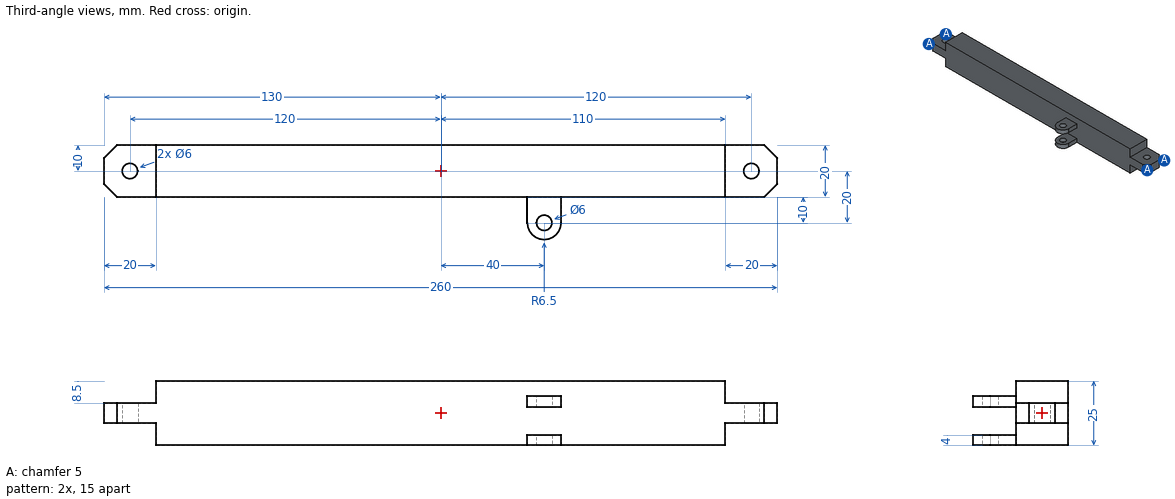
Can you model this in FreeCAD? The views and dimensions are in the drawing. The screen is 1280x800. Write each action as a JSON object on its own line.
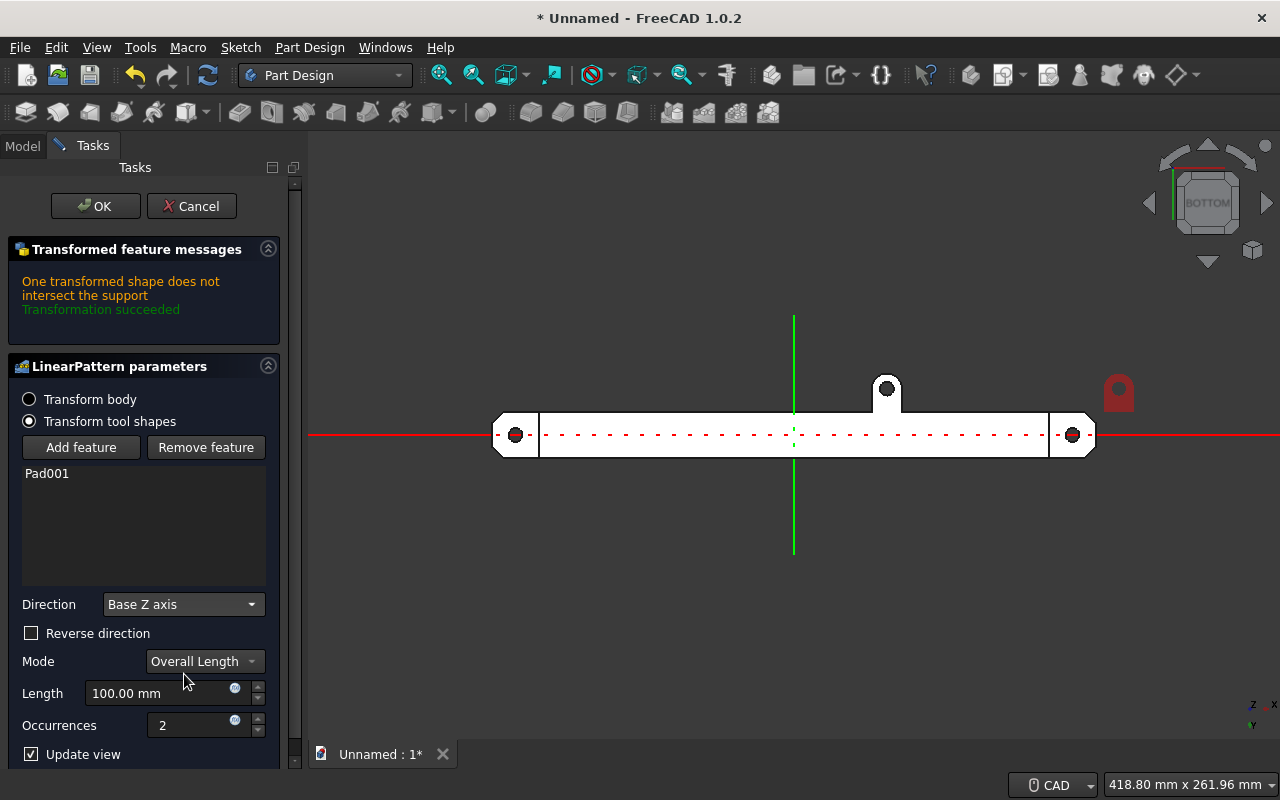
{"action": "left_click", "coordinate": [206, 662]}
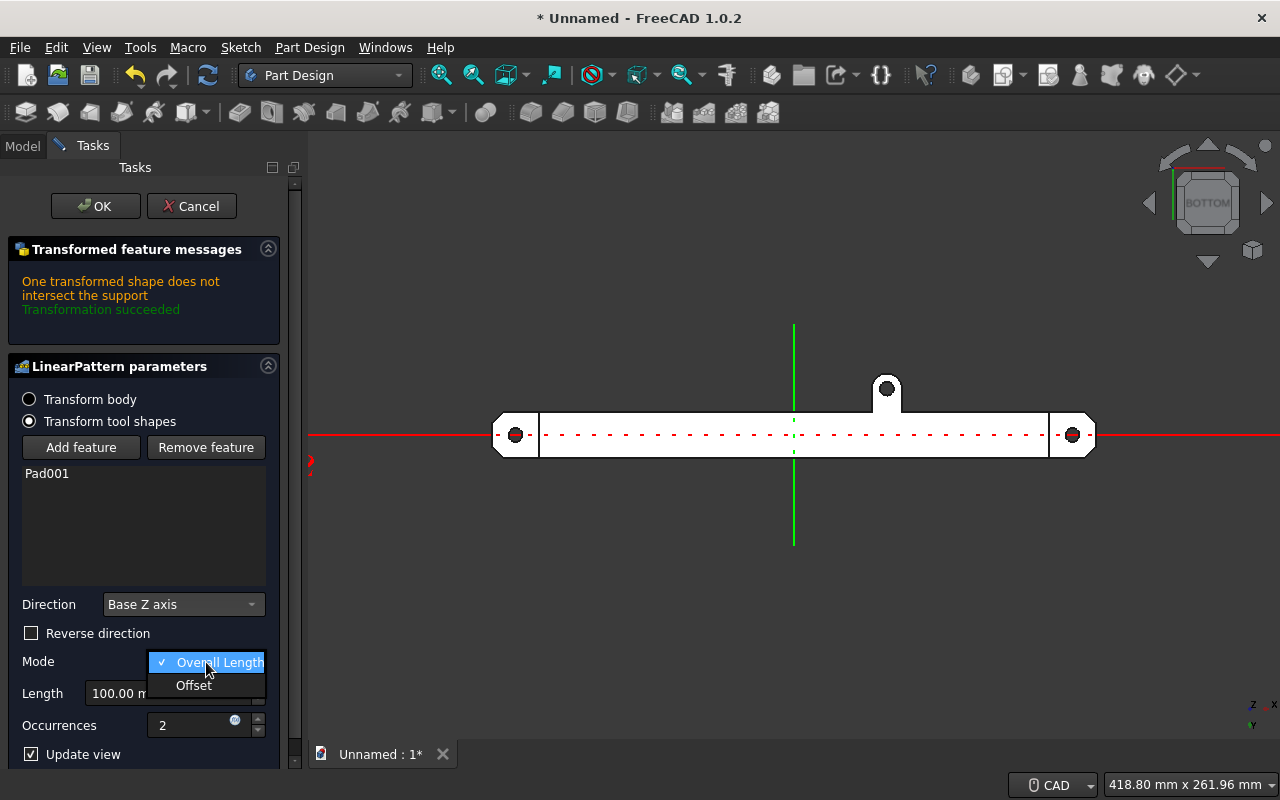
{"action": "left_click", "coordinate": [206, 686]}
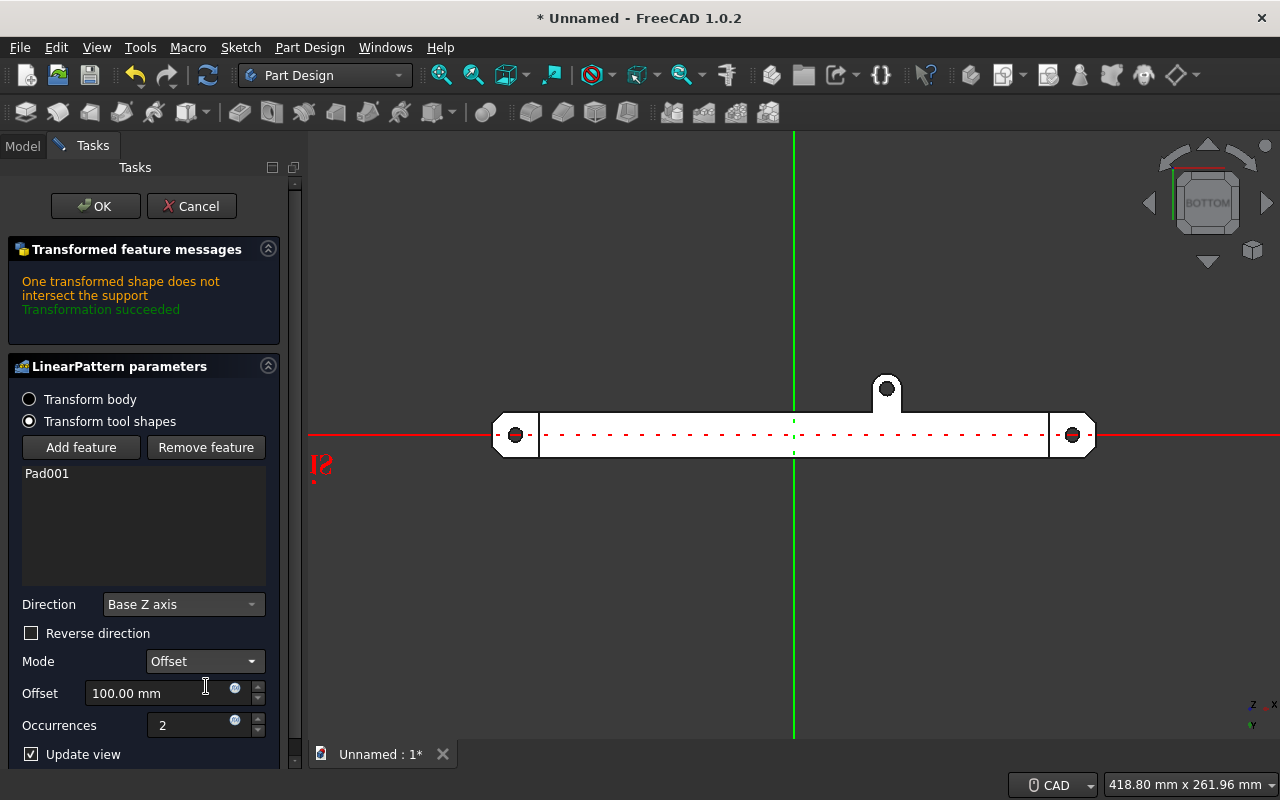
{"action": "triple_click", "coordinate": [168, 693]}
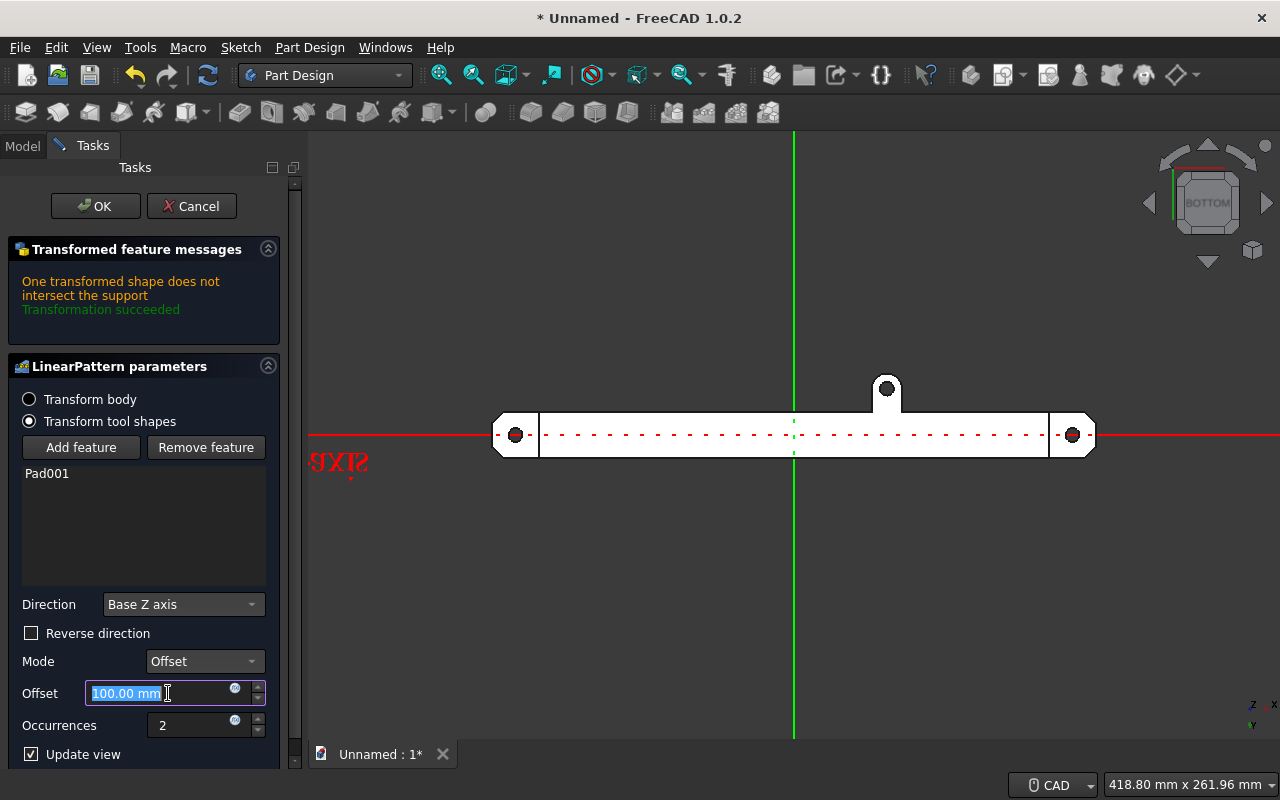
{"action": "type", "text": "15"}
{"action": "key", "text": "Tab"}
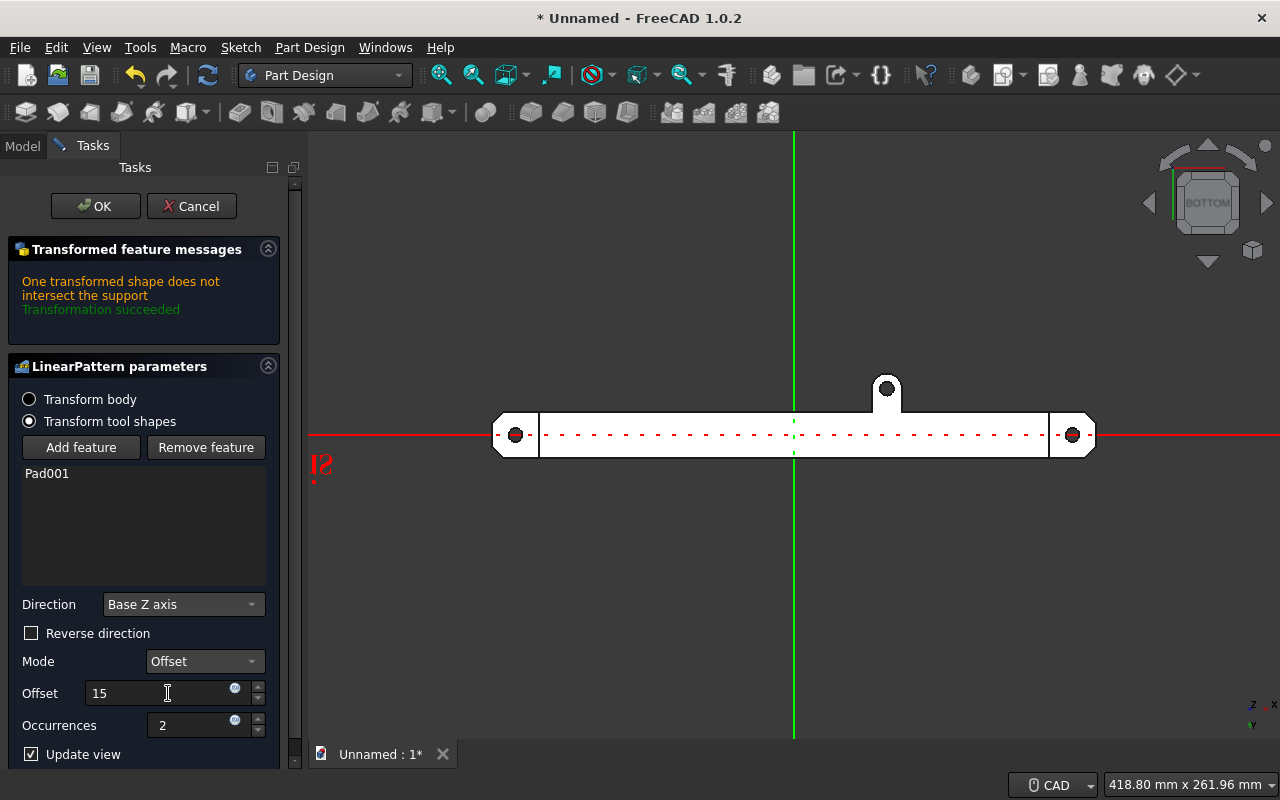
{"action": "triple_click", "coordinate": [198, 725]}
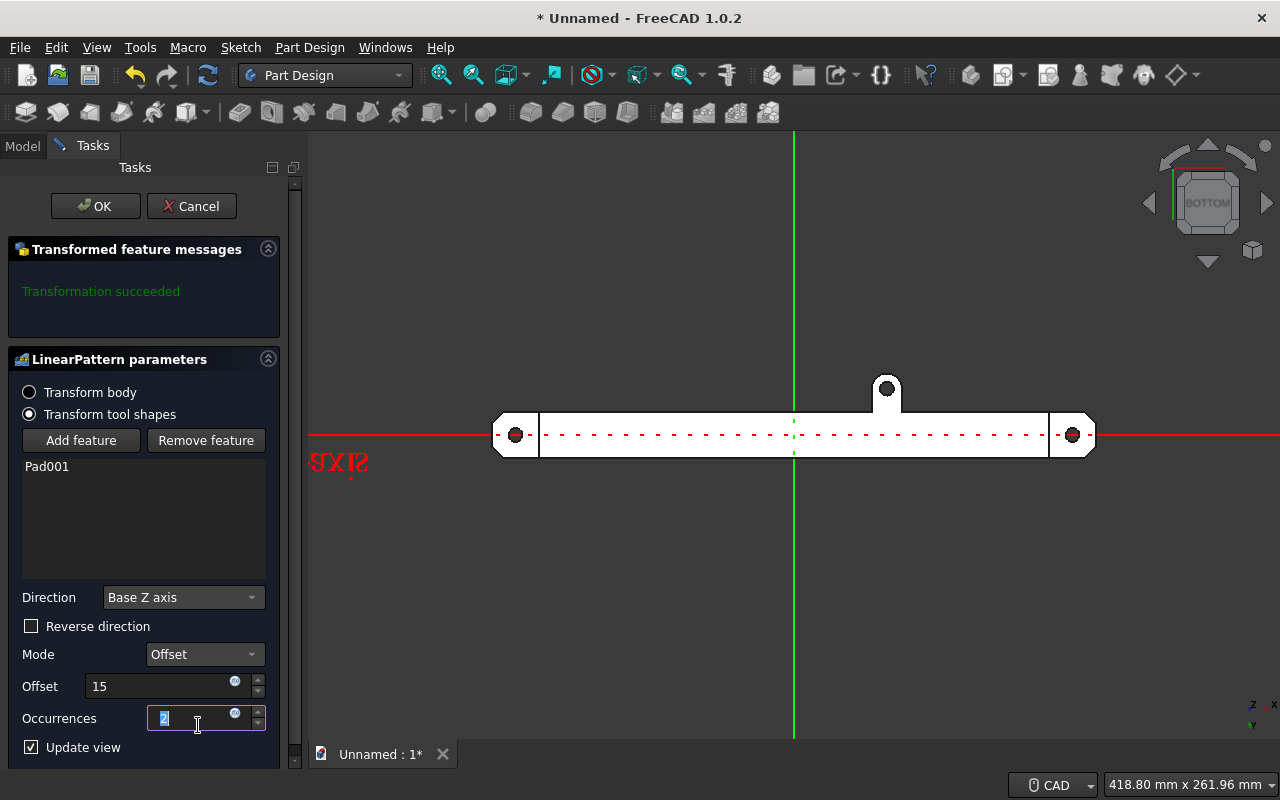
{"action": "type", "text": "2"}
{"action": "key", "text": "Tab"}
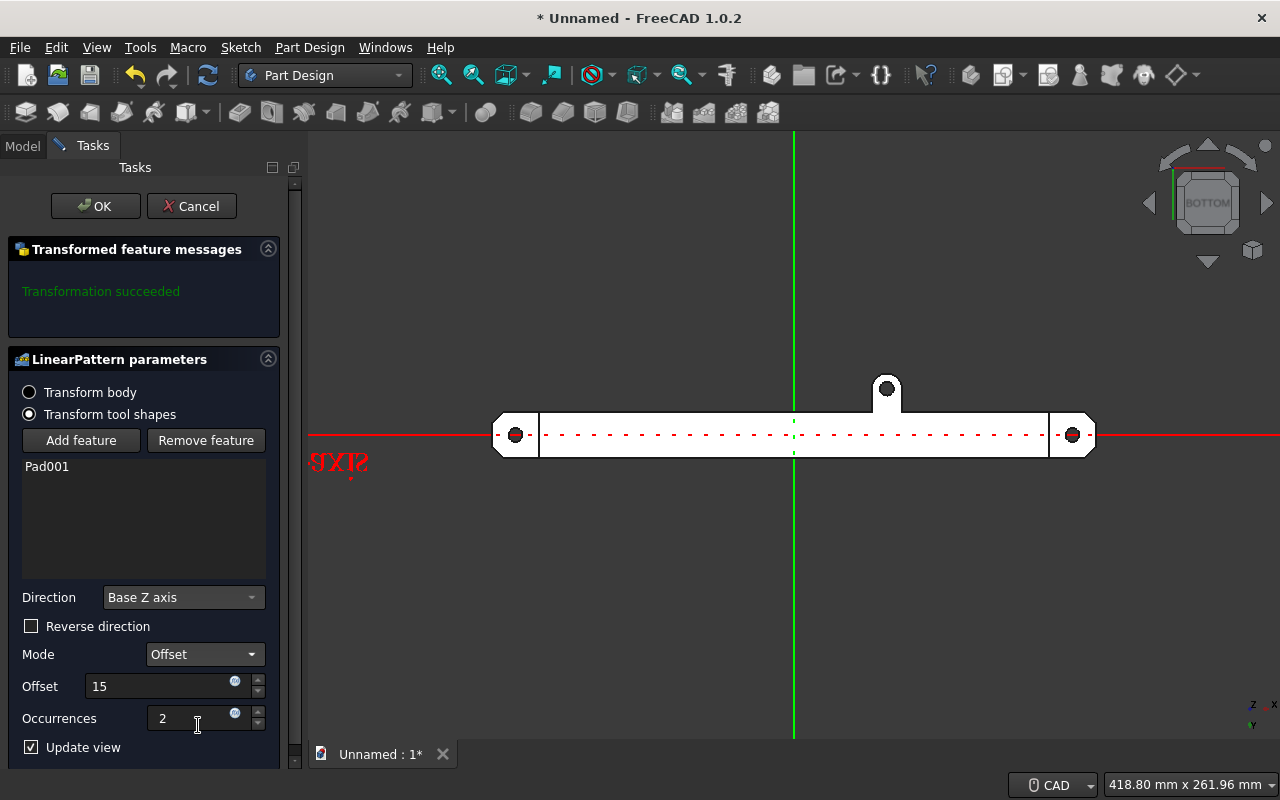
{"action": "left_click", "coordinate": [96, 206]}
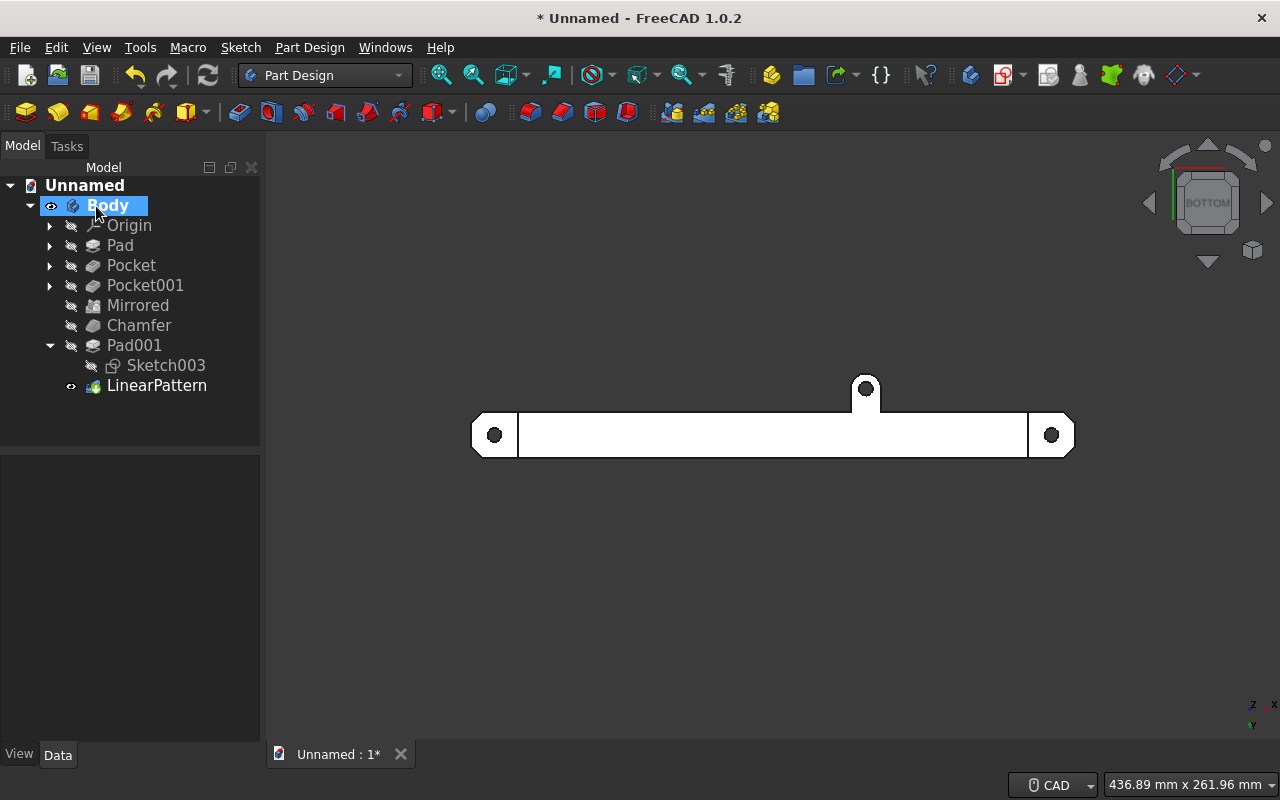
{"action": "key", "text": "0"}